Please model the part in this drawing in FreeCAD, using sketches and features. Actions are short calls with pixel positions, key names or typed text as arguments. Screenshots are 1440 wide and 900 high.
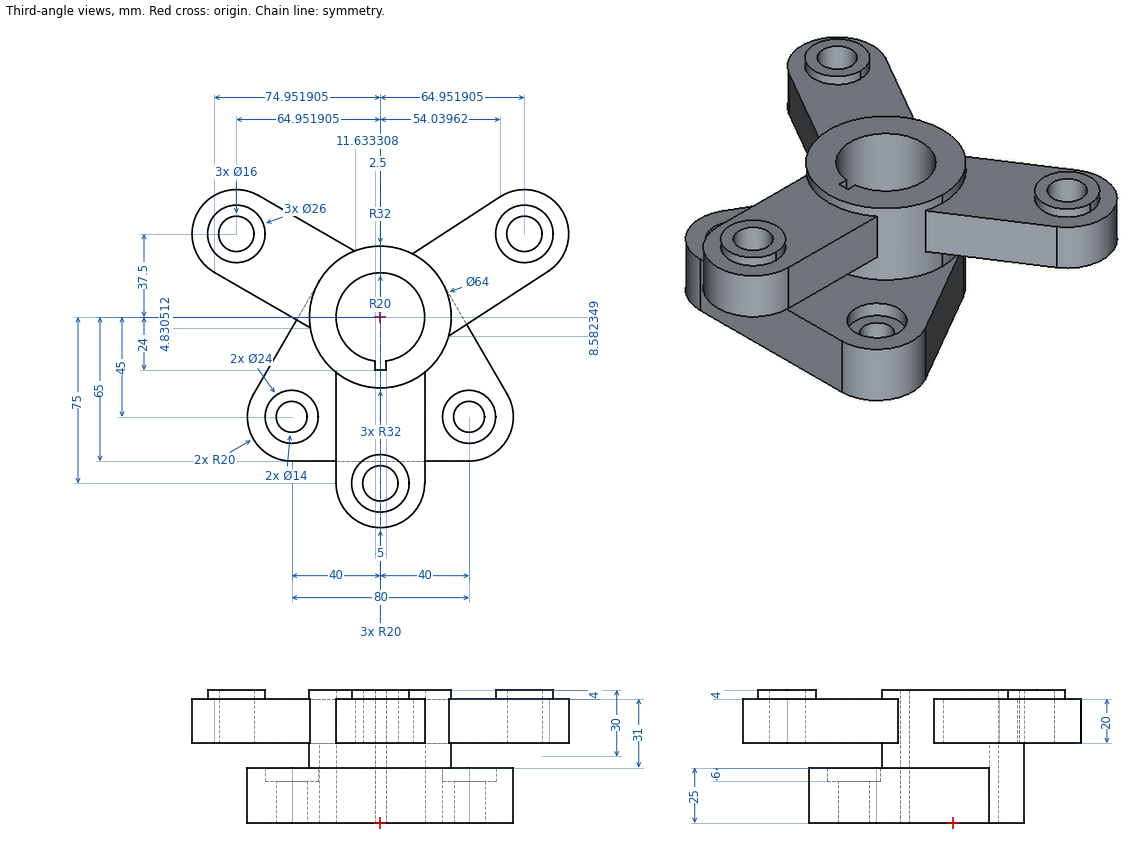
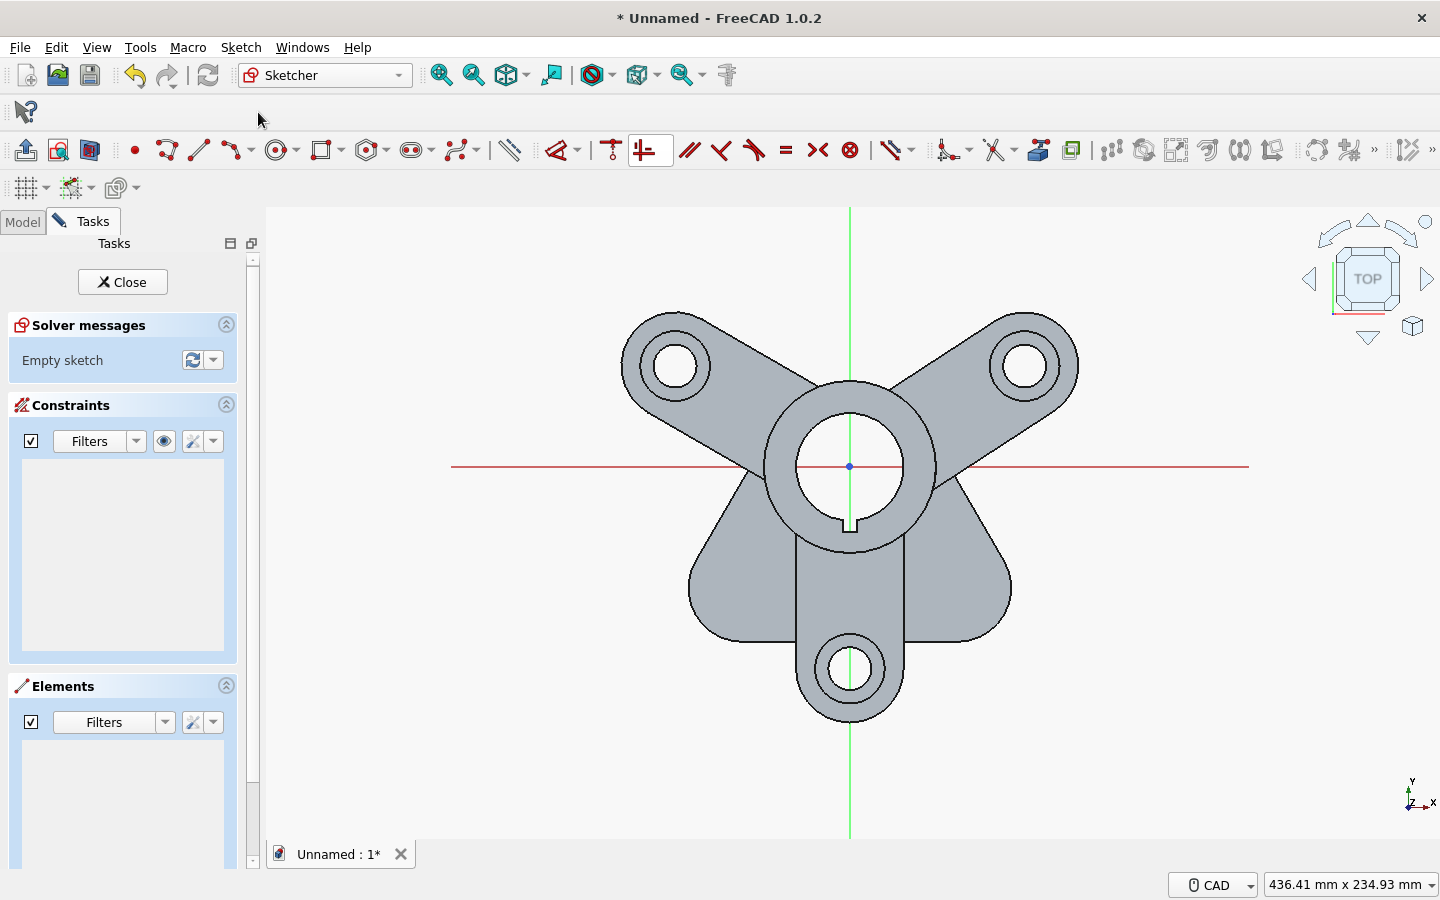
click(90, 150)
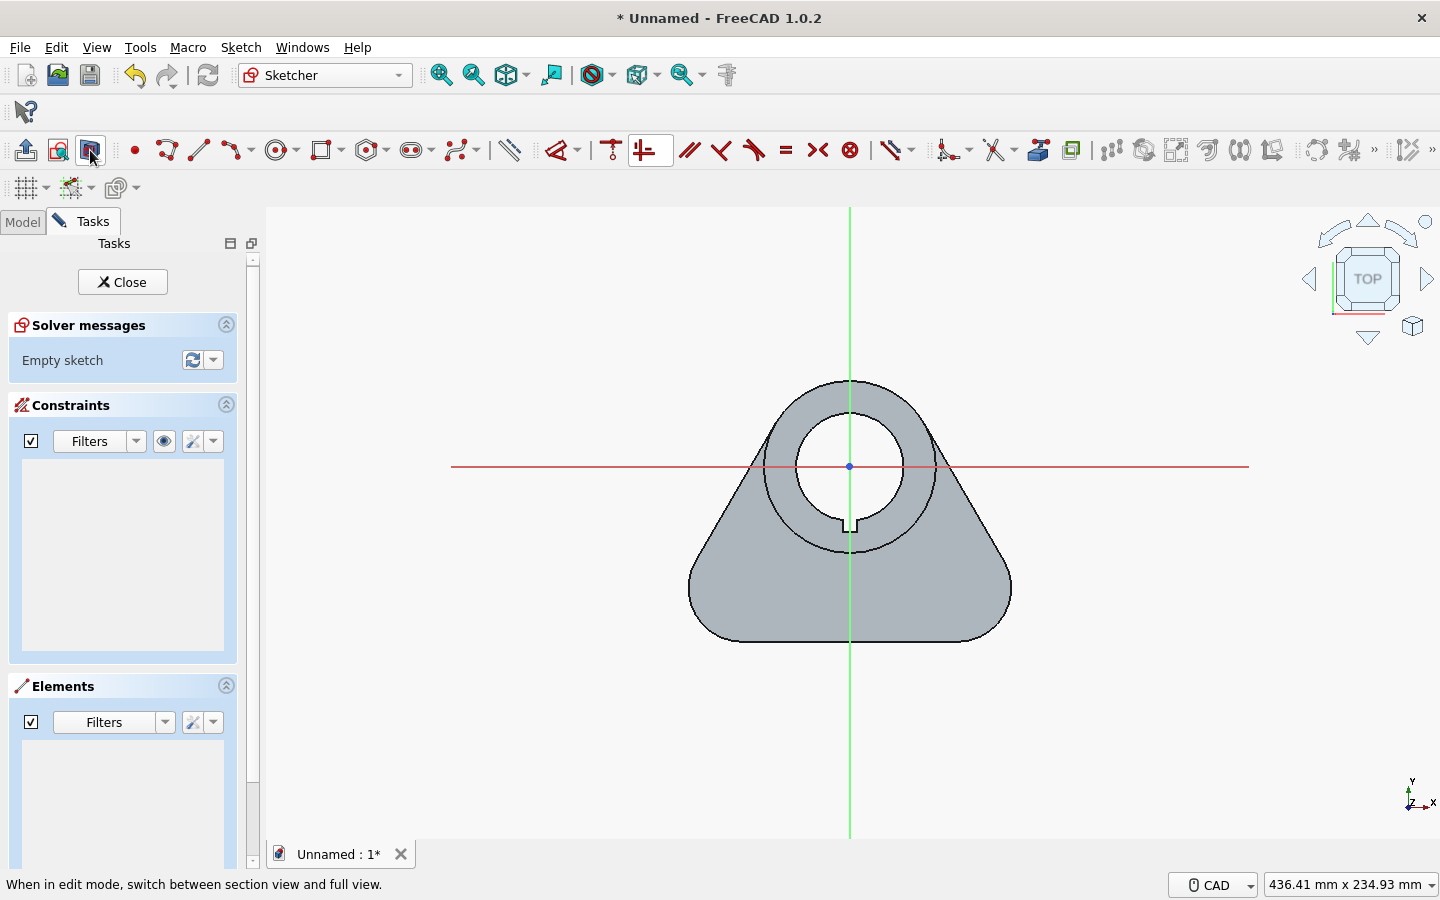
scroll(888, 556, up, 5)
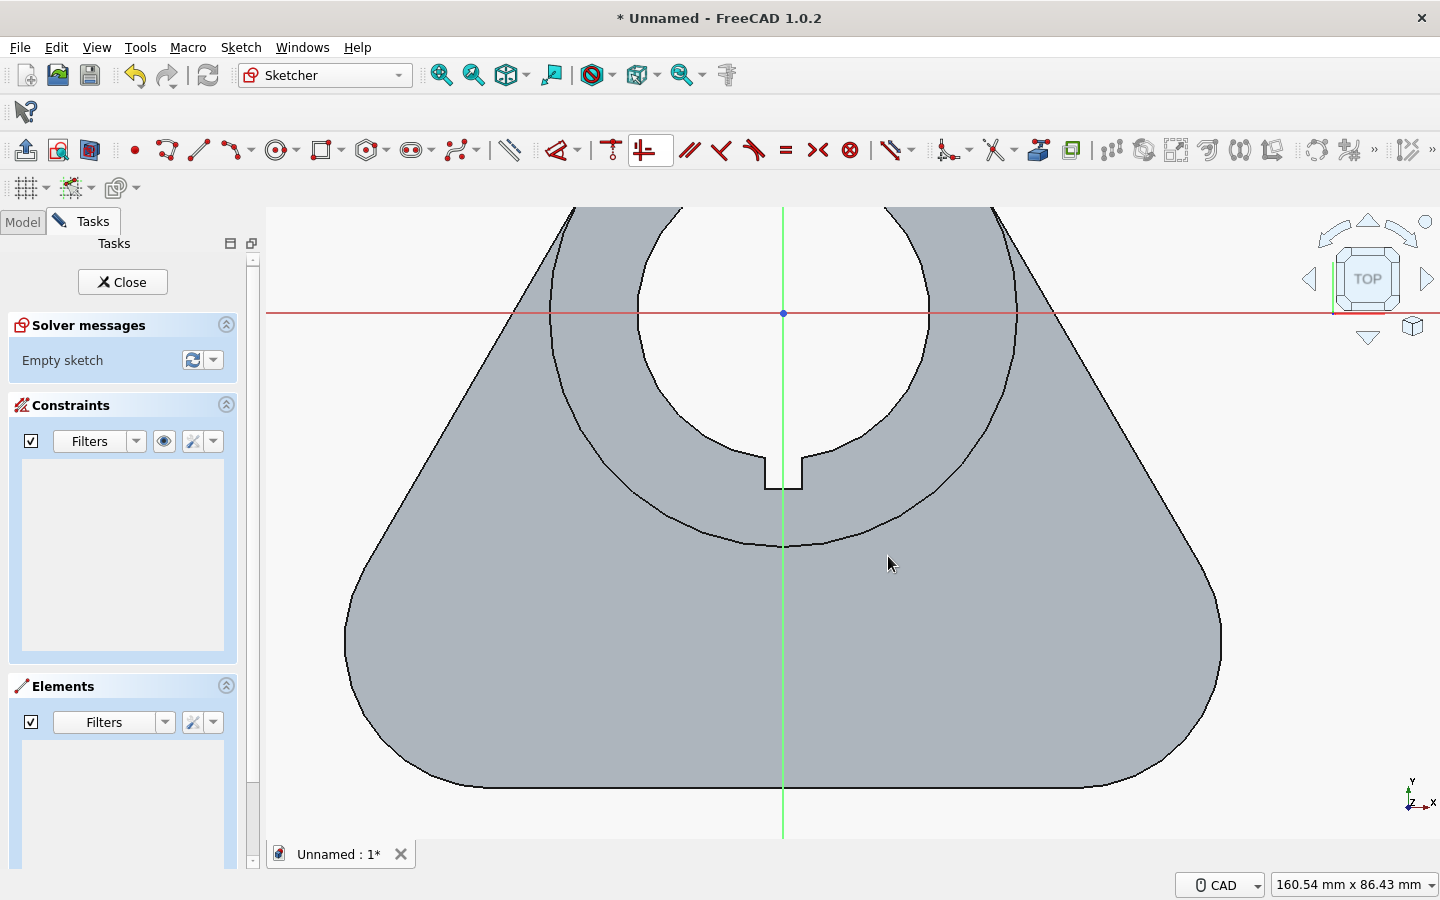
click(276, 150)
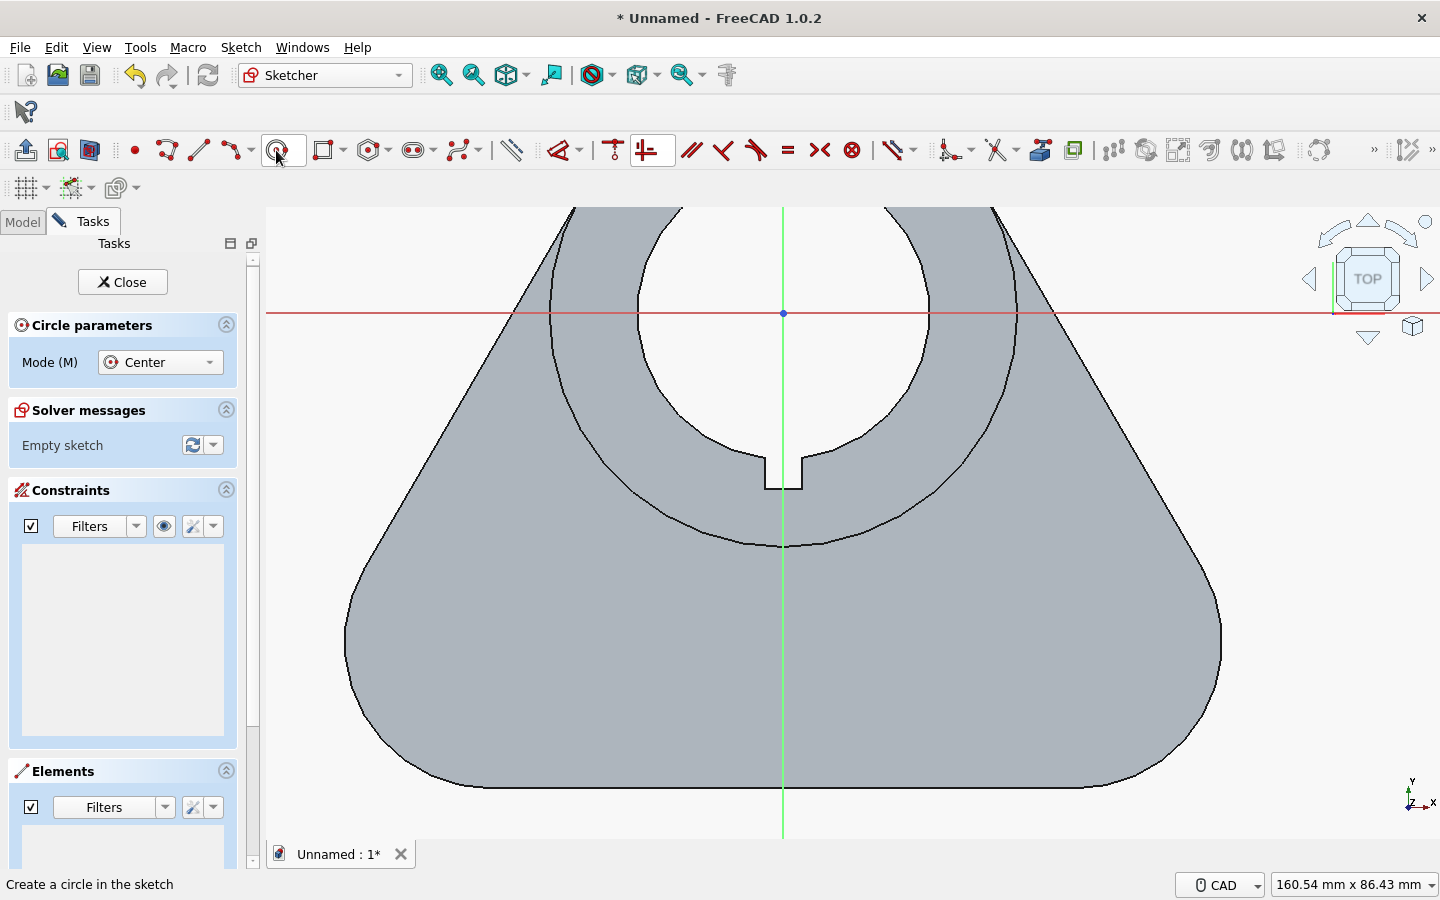
click(491, 642)
move(553, 580)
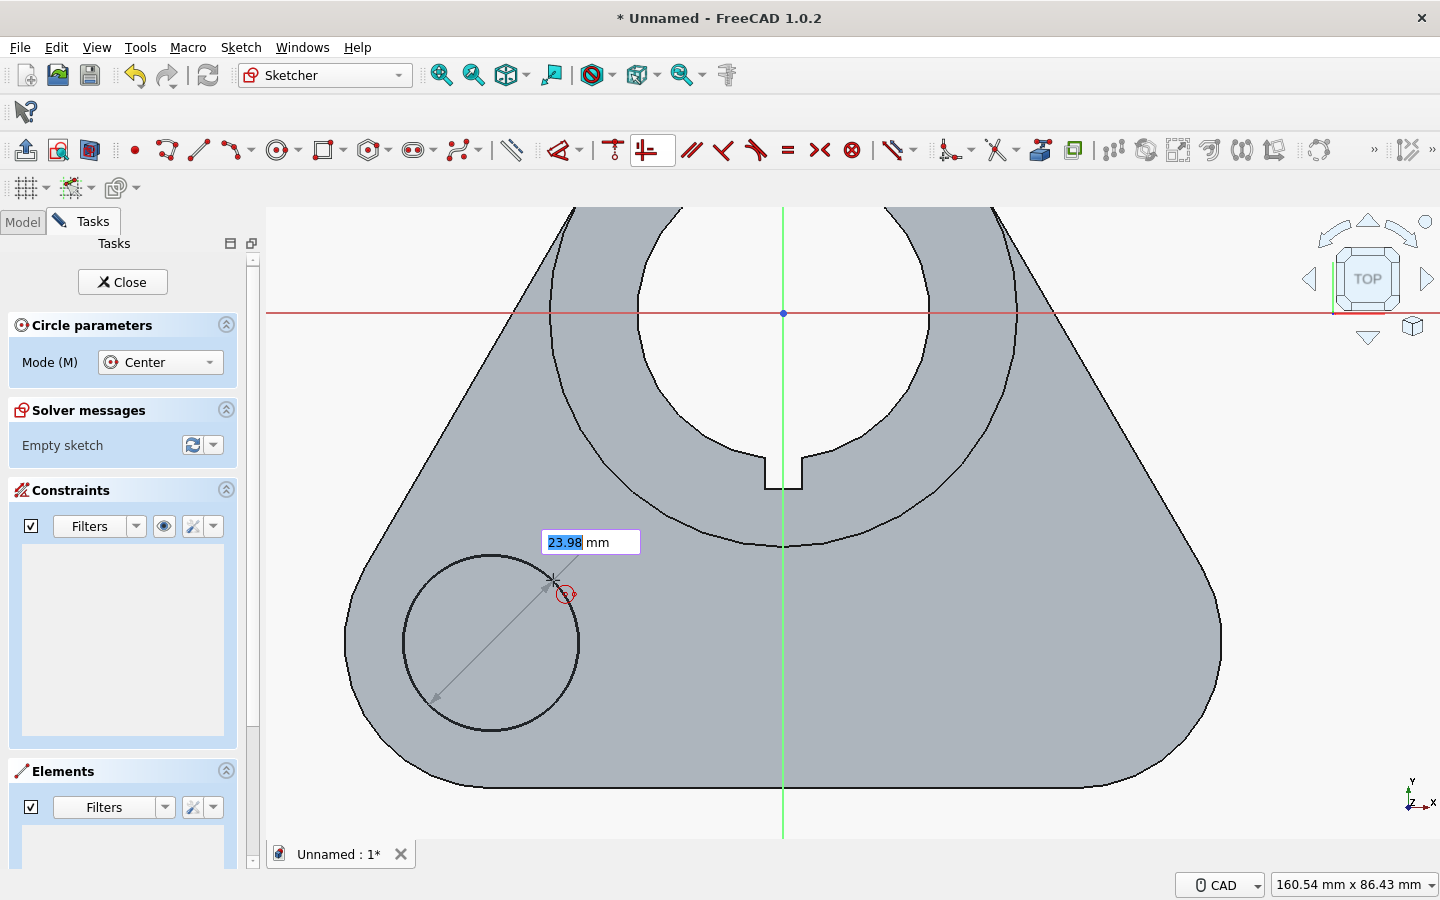
text(24)
key(Return)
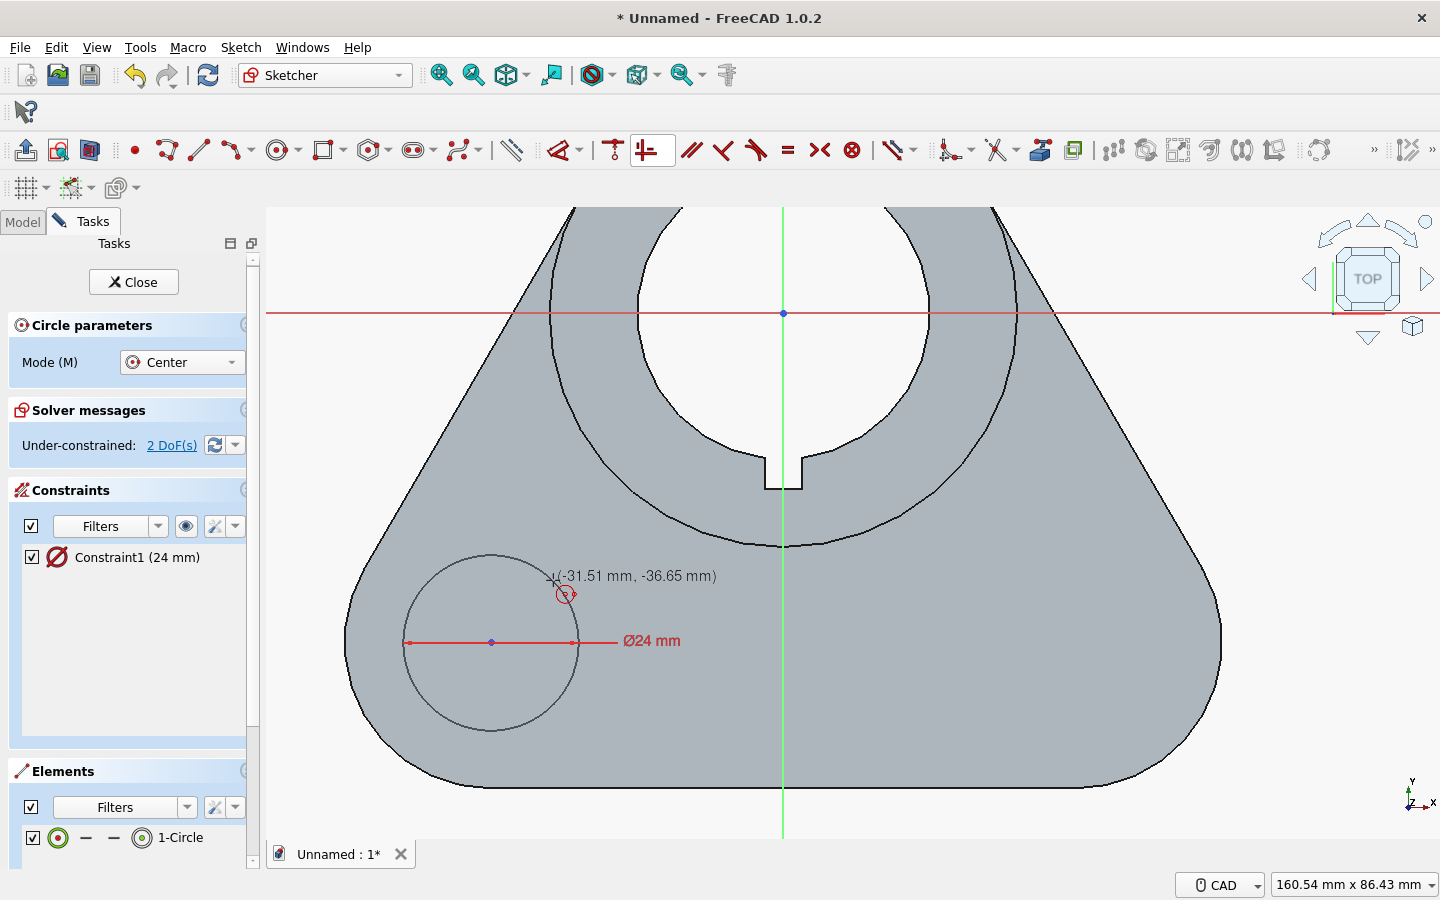
click(1076, 642)
move(1138, 580)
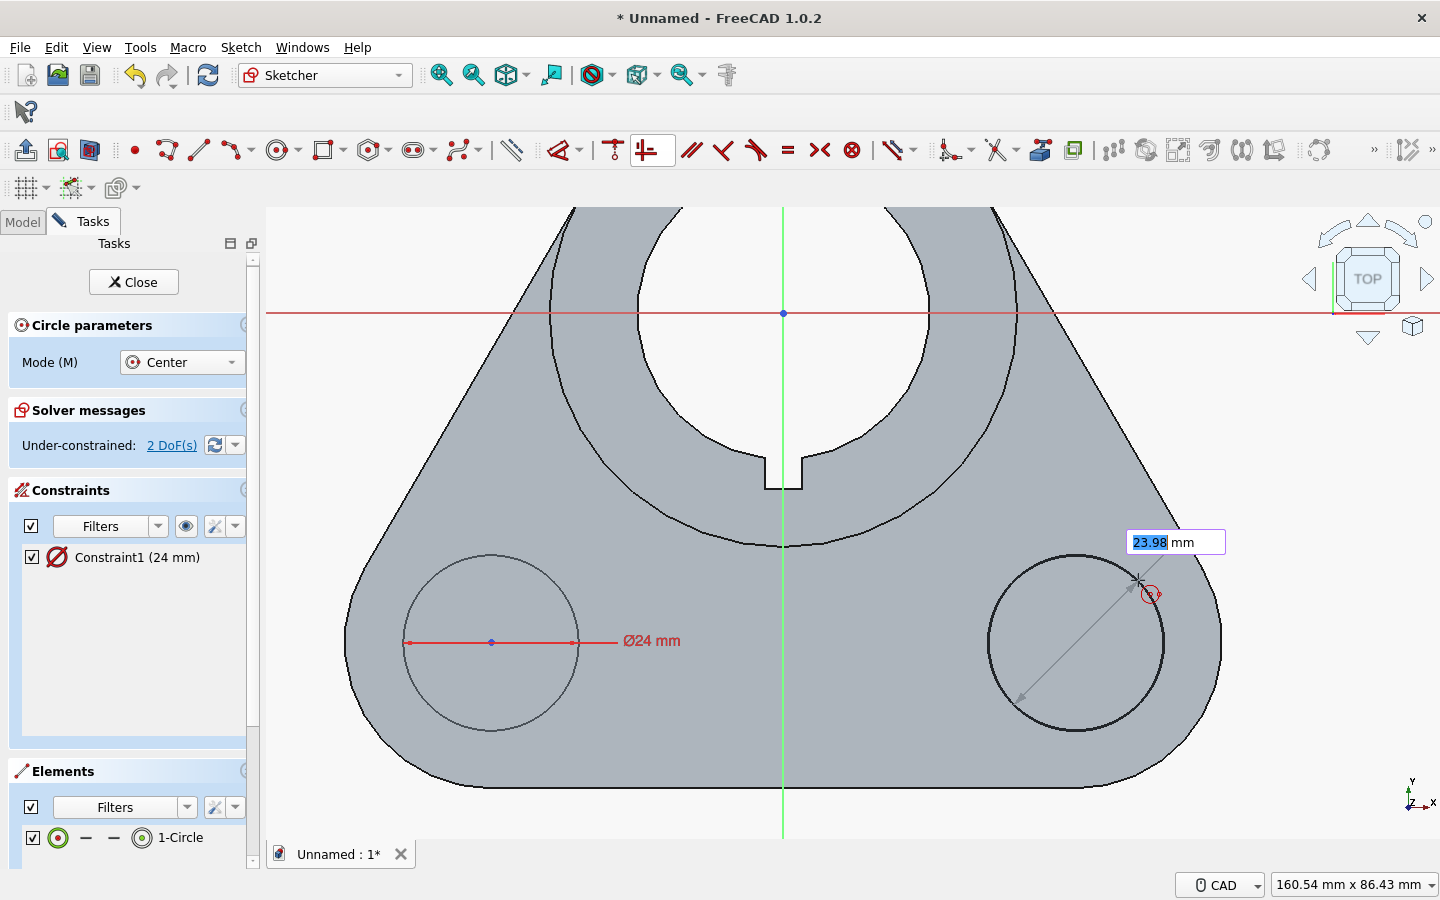
text(24)
key(Return)
key(Escape)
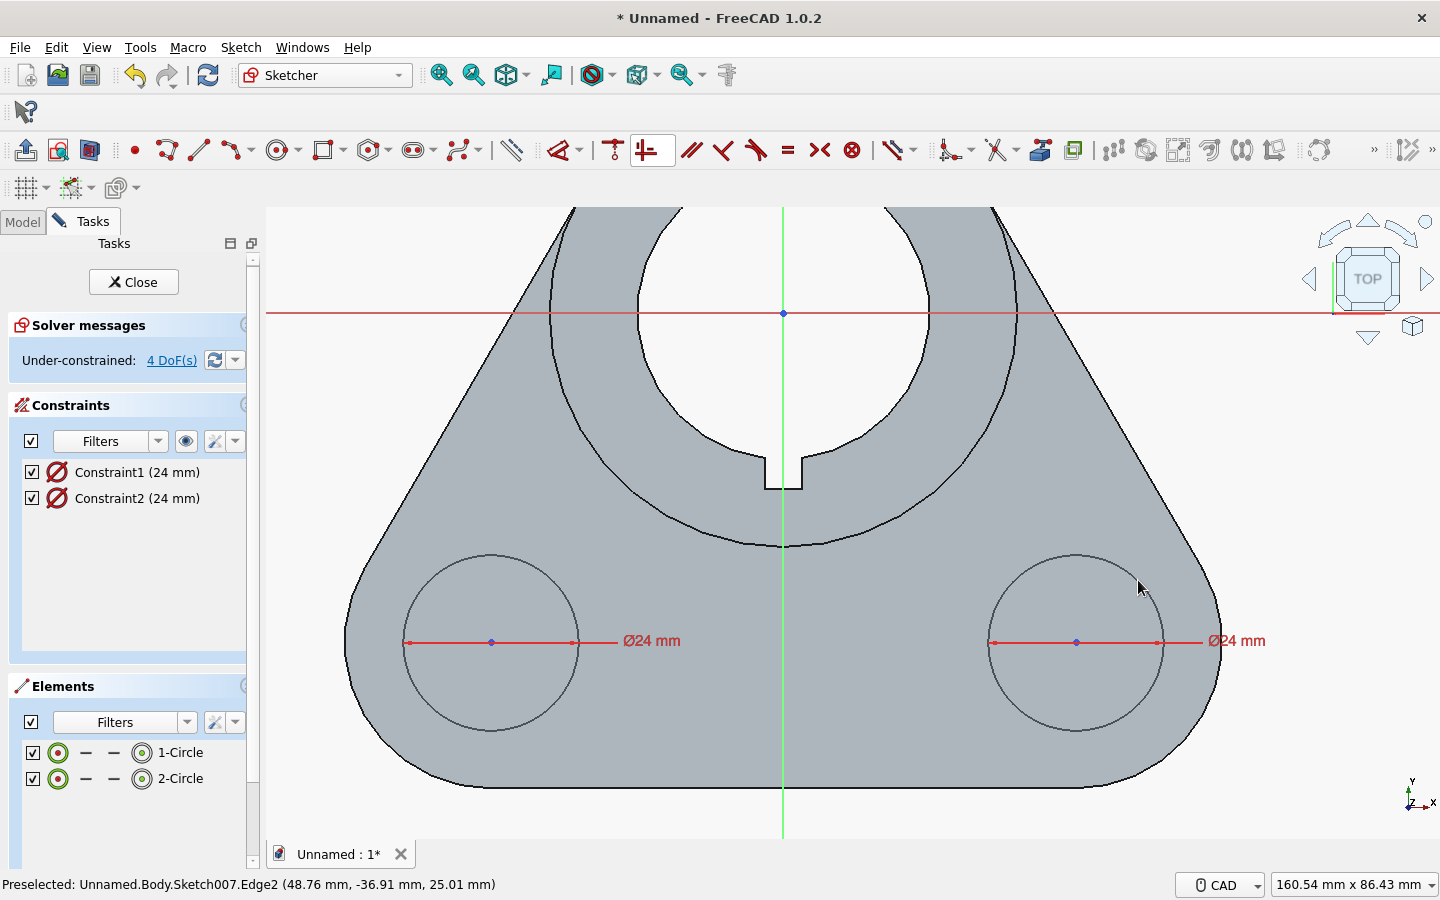
click(491, 643)